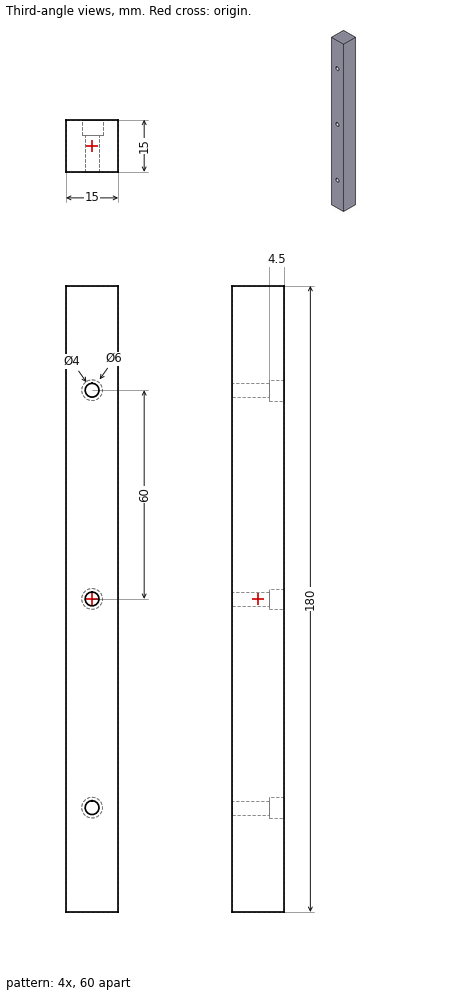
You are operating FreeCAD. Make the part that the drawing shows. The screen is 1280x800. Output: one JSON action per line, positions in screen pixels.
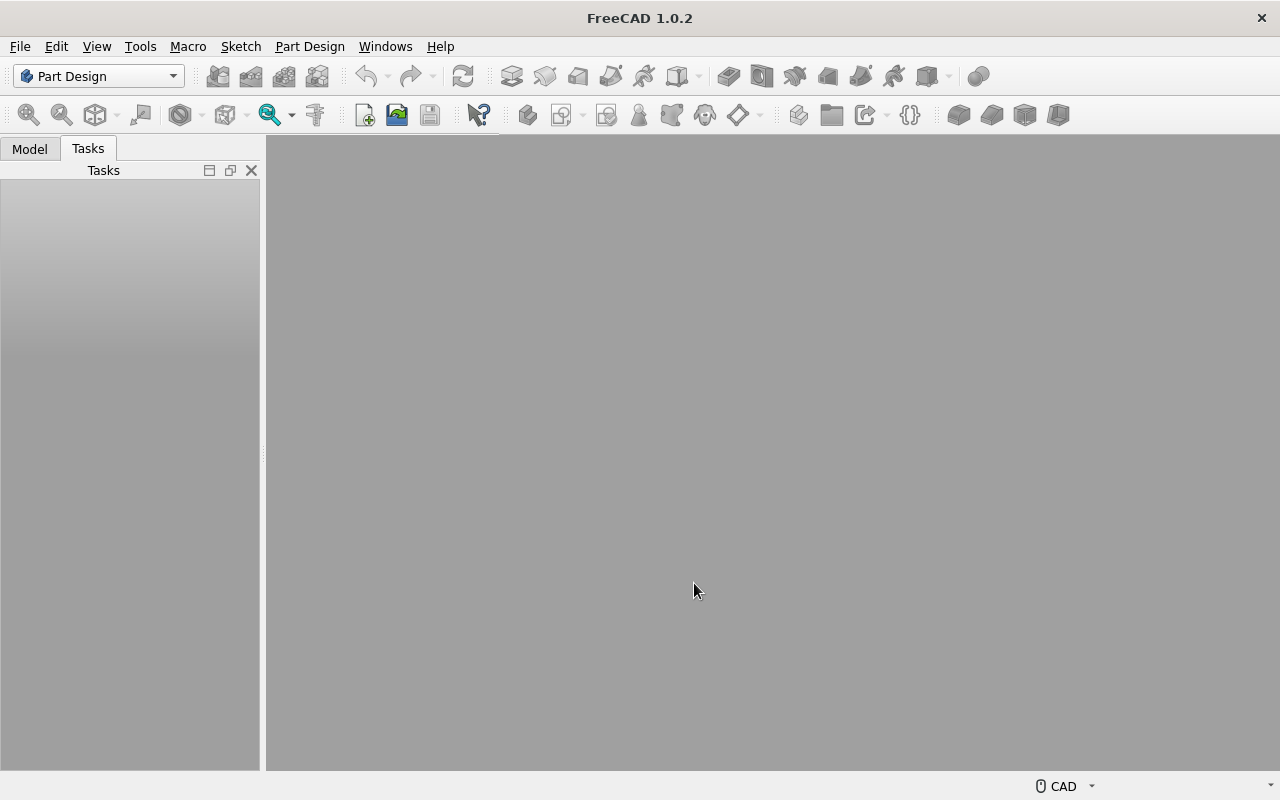
{"action": "left_click", "coordinate": [364, 116]}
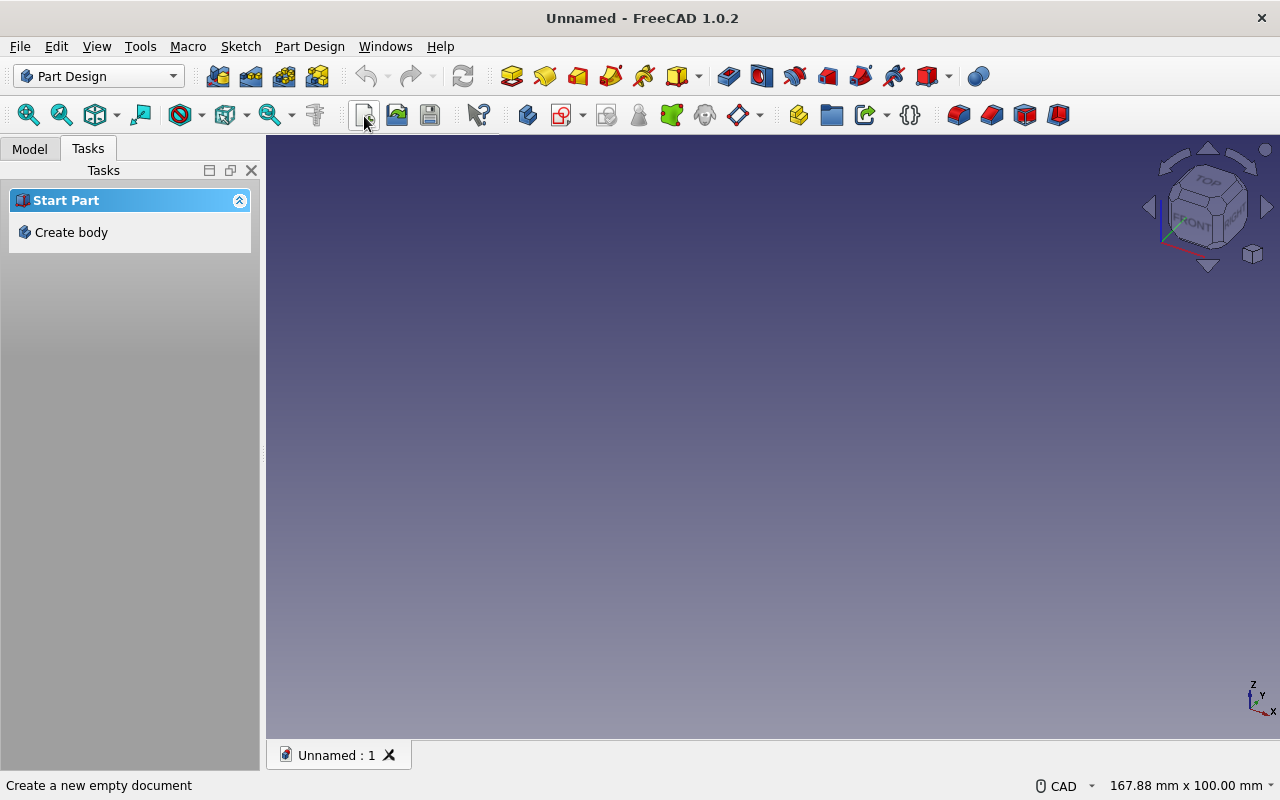
{"action": "left_click", "coordinate": [560, 116]}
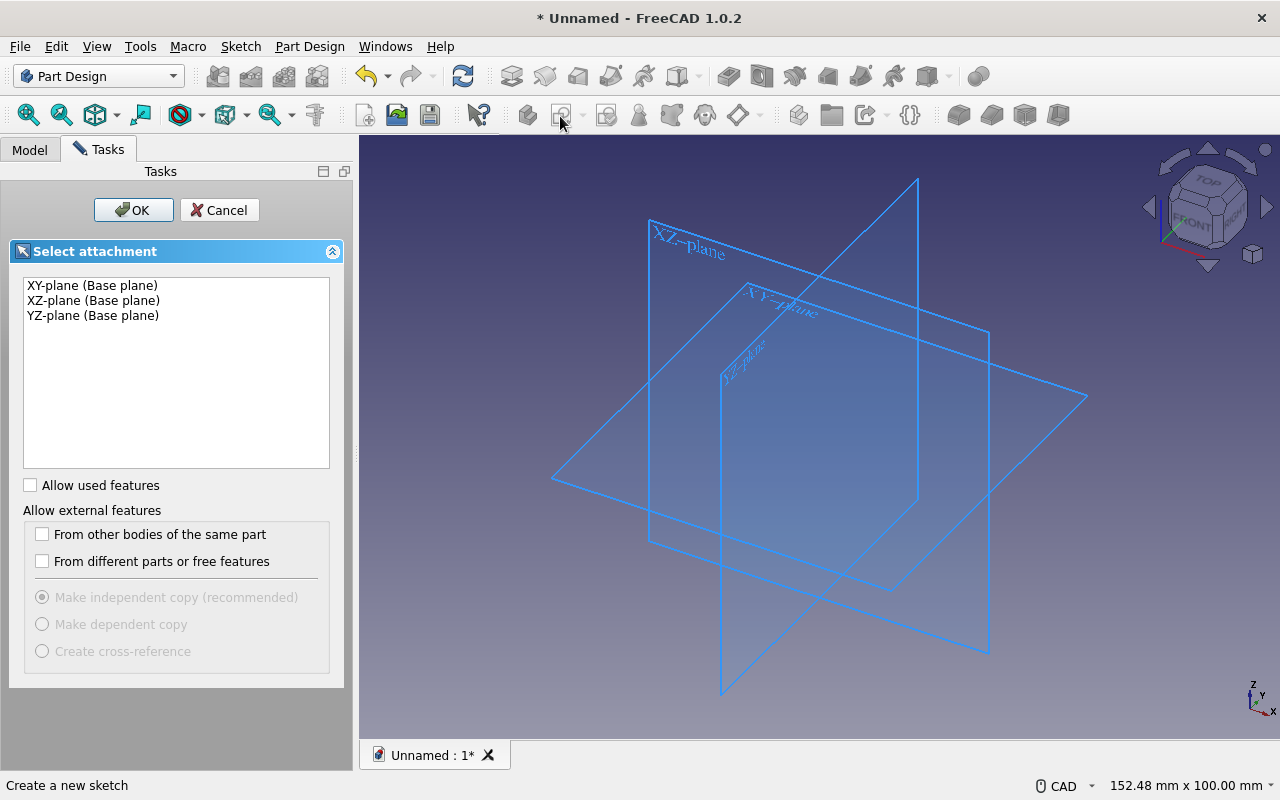
{"action": "left_click", "coordinate": [84, 286]}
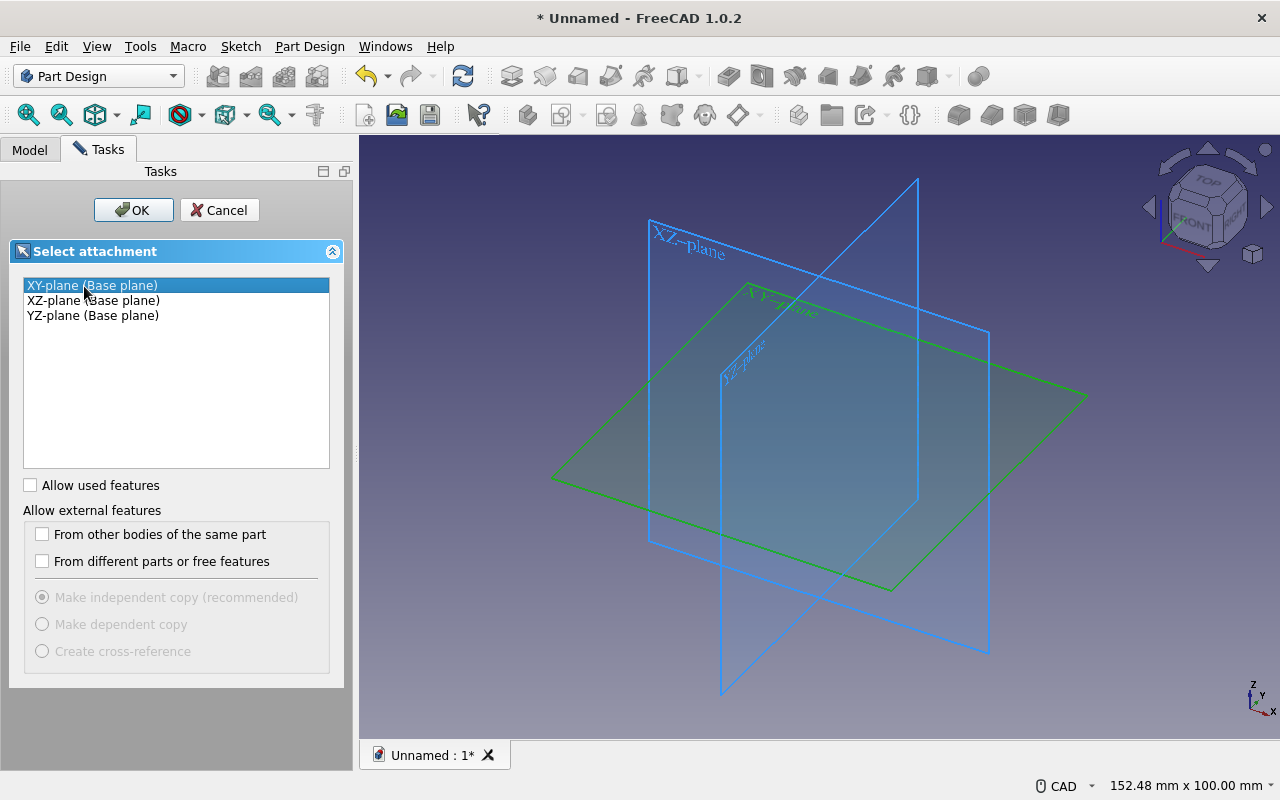
{"action": "left_click", "coordinate": [134, 210]}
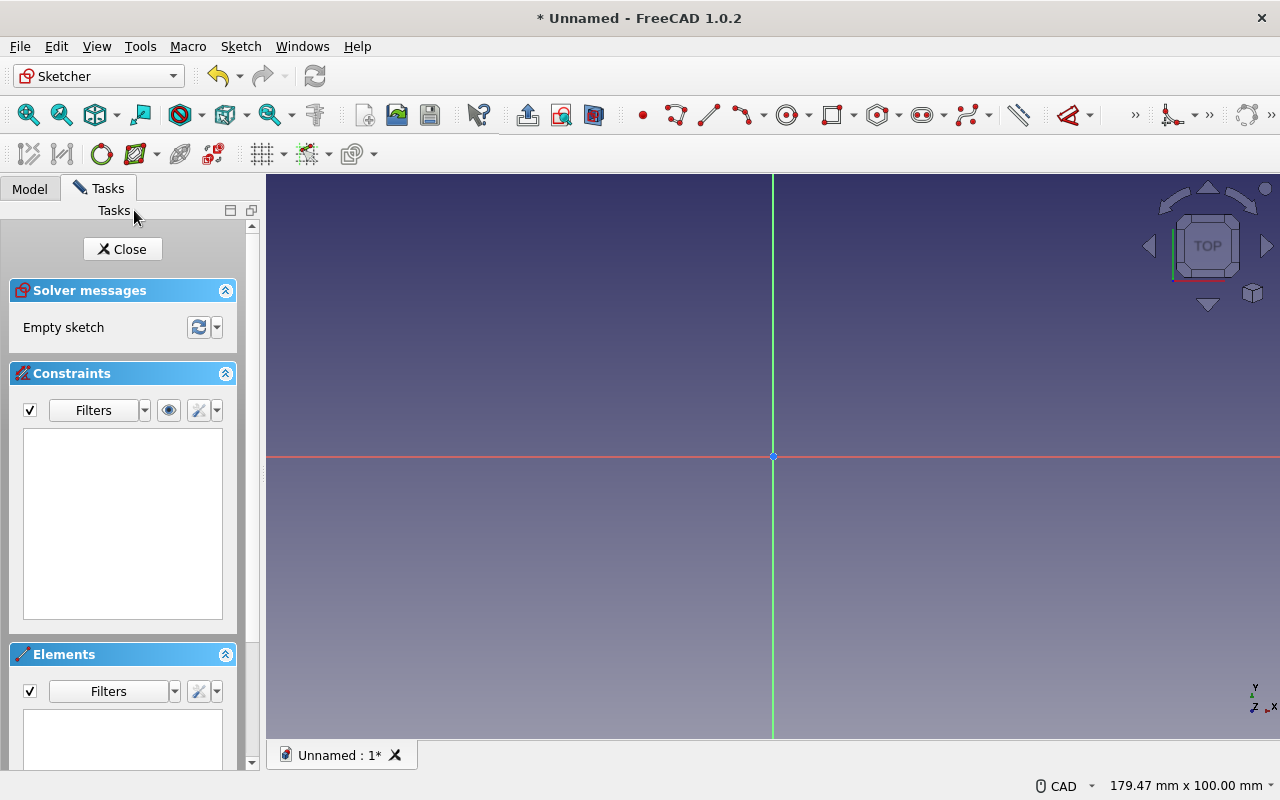
{"action": "scroll", "coordinate": [795, 456], "scroll_direction": "up", "scroll_amount": 7}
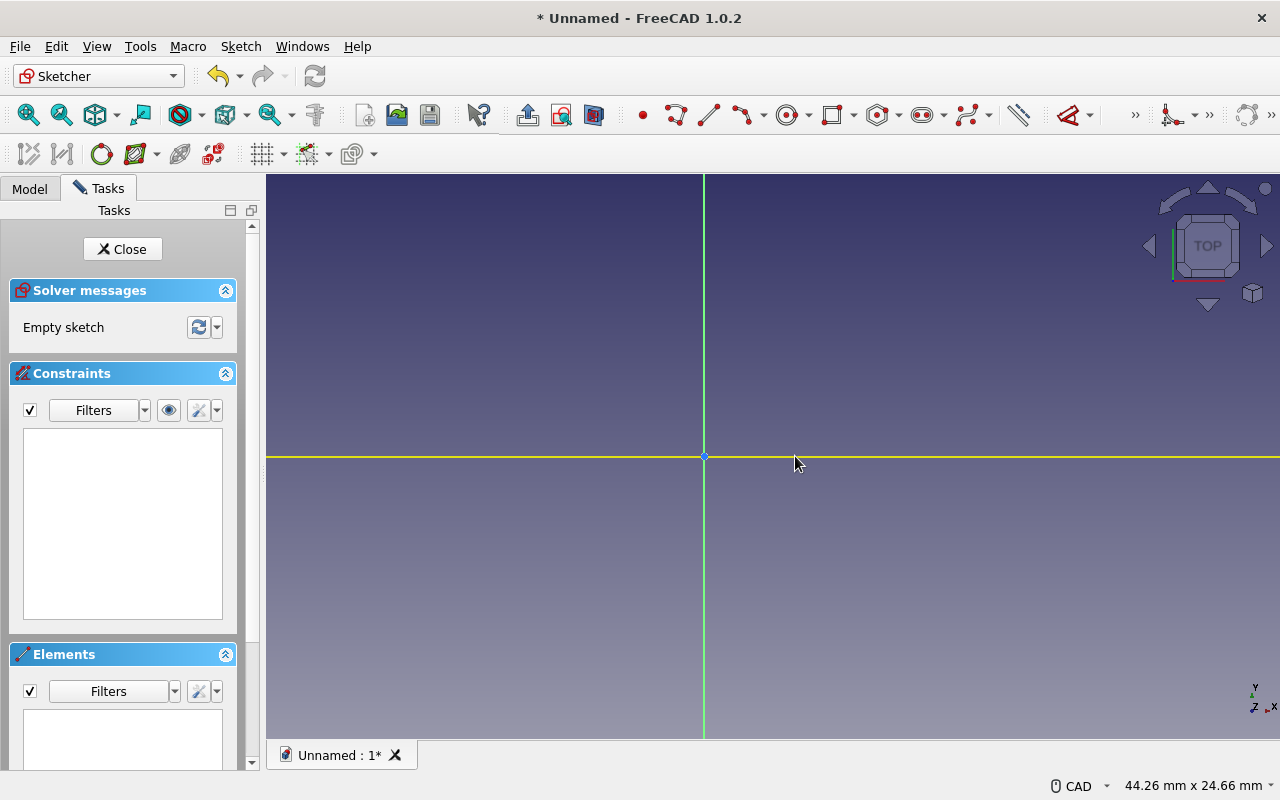
{"action": "left_click", "coordinate": [854, 116]}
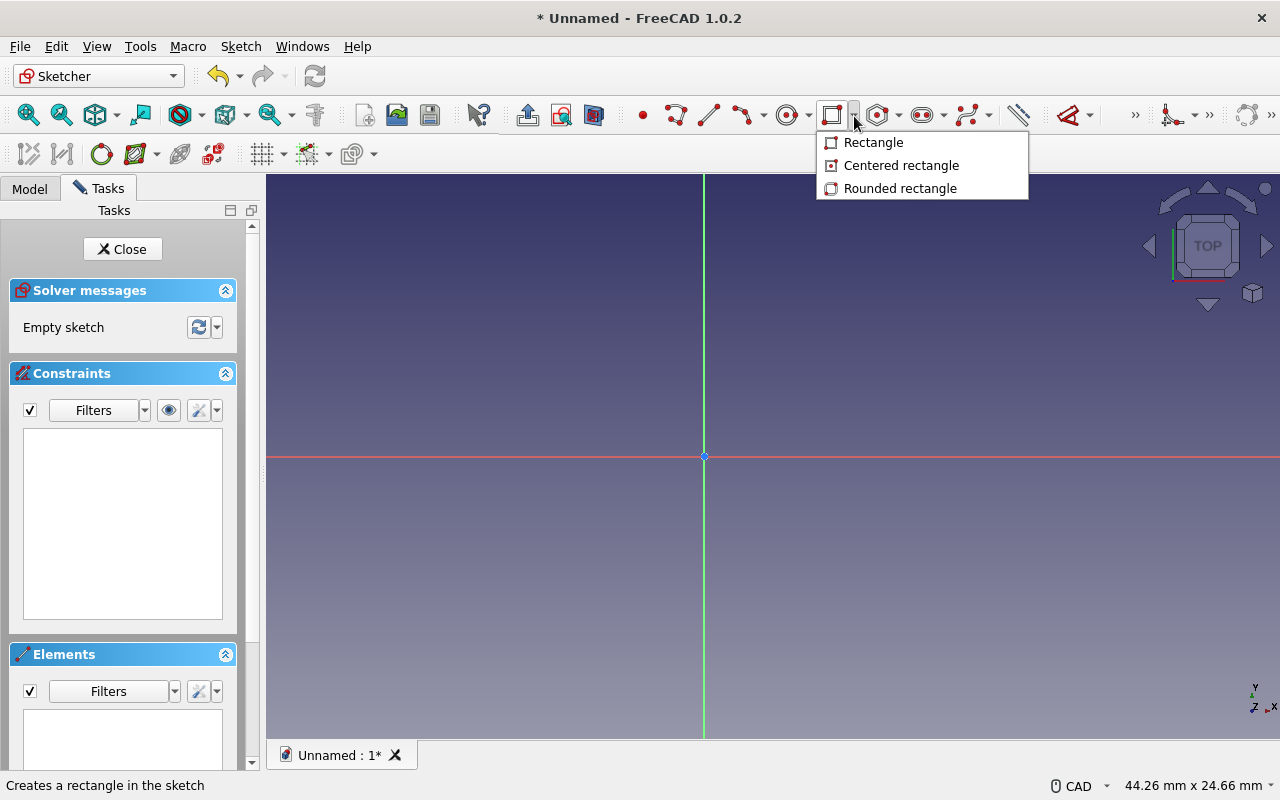
{"action": "left_click", "coordinate": [922, 166]}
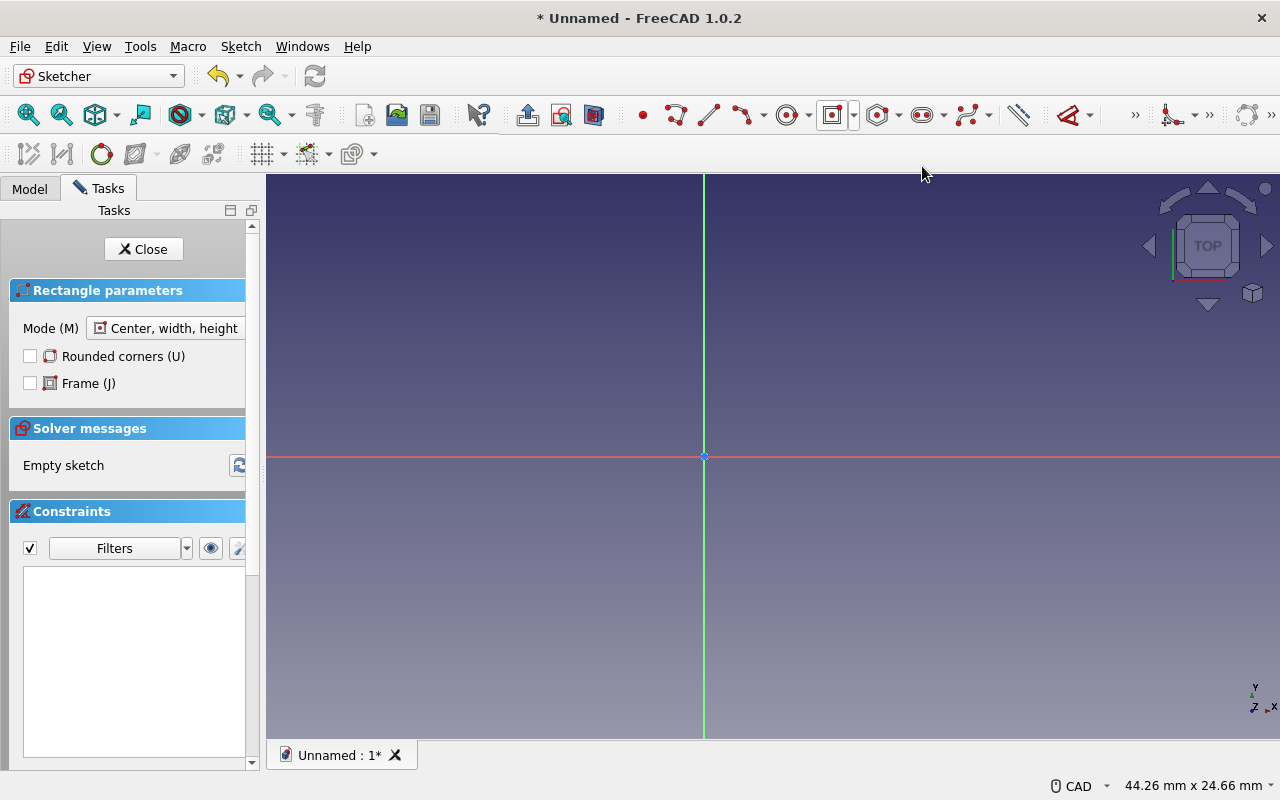
{"action": "left_click", "coordinate": [704, 456]}
{"action": "mouse_move", "coordinate": [876, 285]}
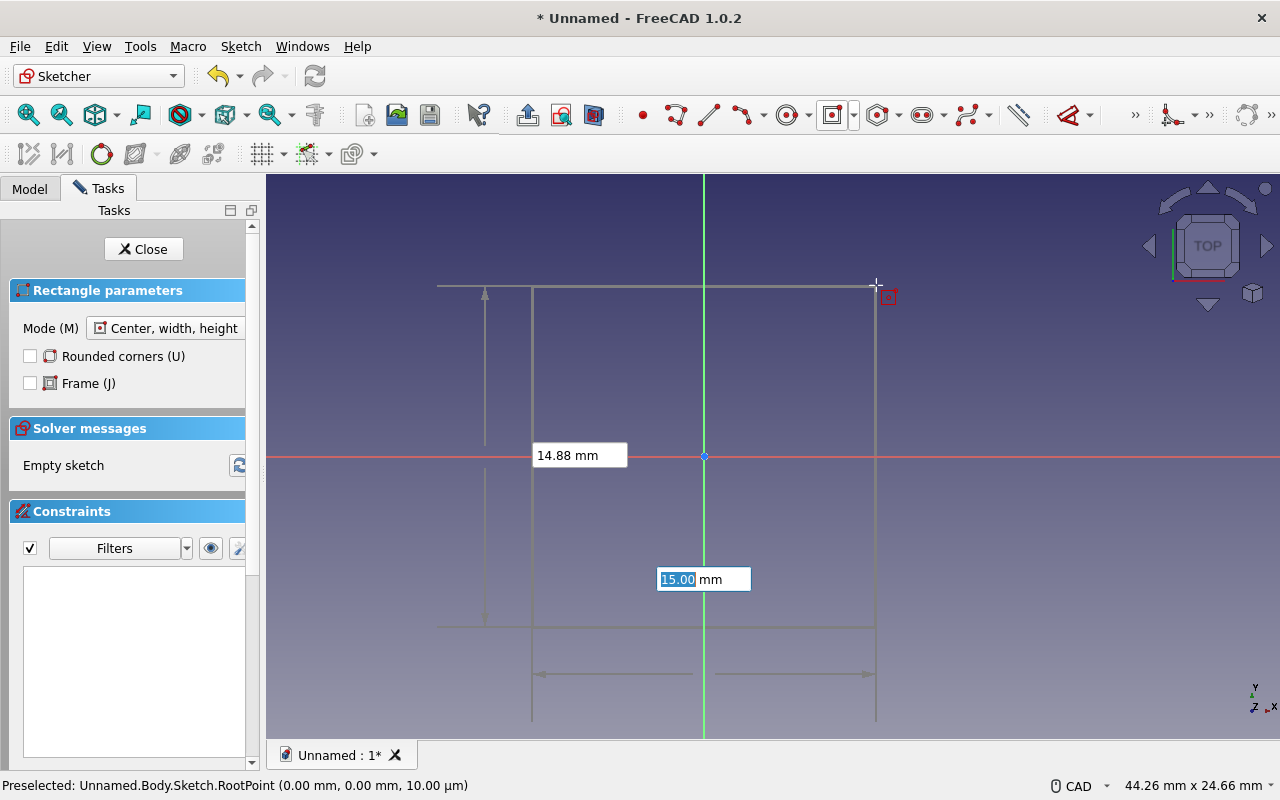
{"action": "type", "text": "15"}
{"action": "key", "text": "Tab"}
{"action": "type", "text": "15"}
{"action": "key", "text": "Return"}
{"action": "key", "text": "Escape"}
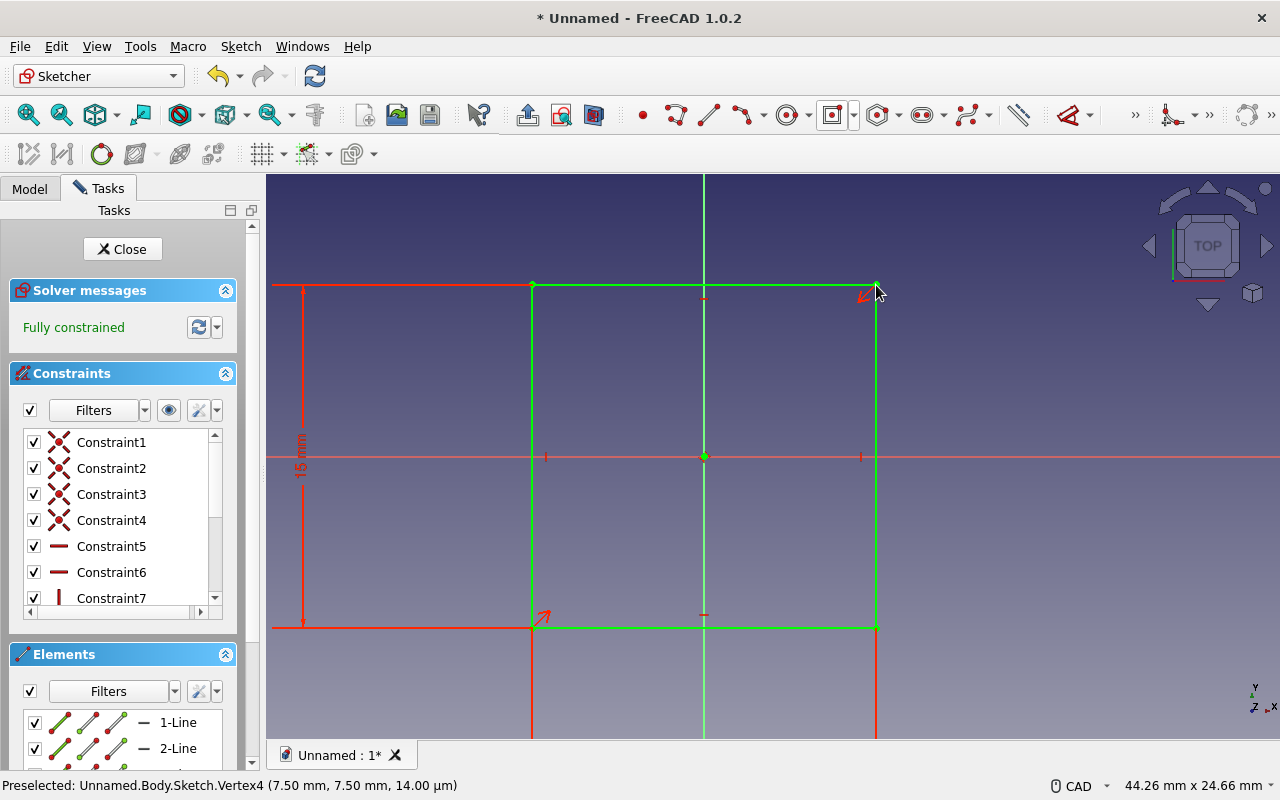
{"action": "left_click", "coordinate": [123, 249]}